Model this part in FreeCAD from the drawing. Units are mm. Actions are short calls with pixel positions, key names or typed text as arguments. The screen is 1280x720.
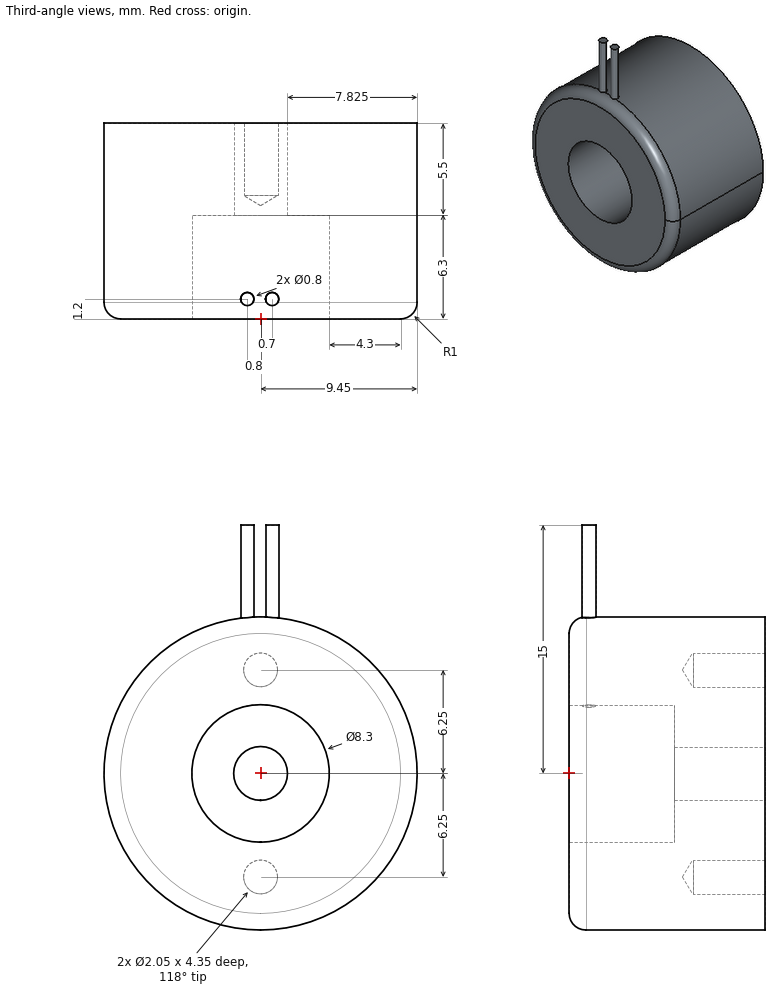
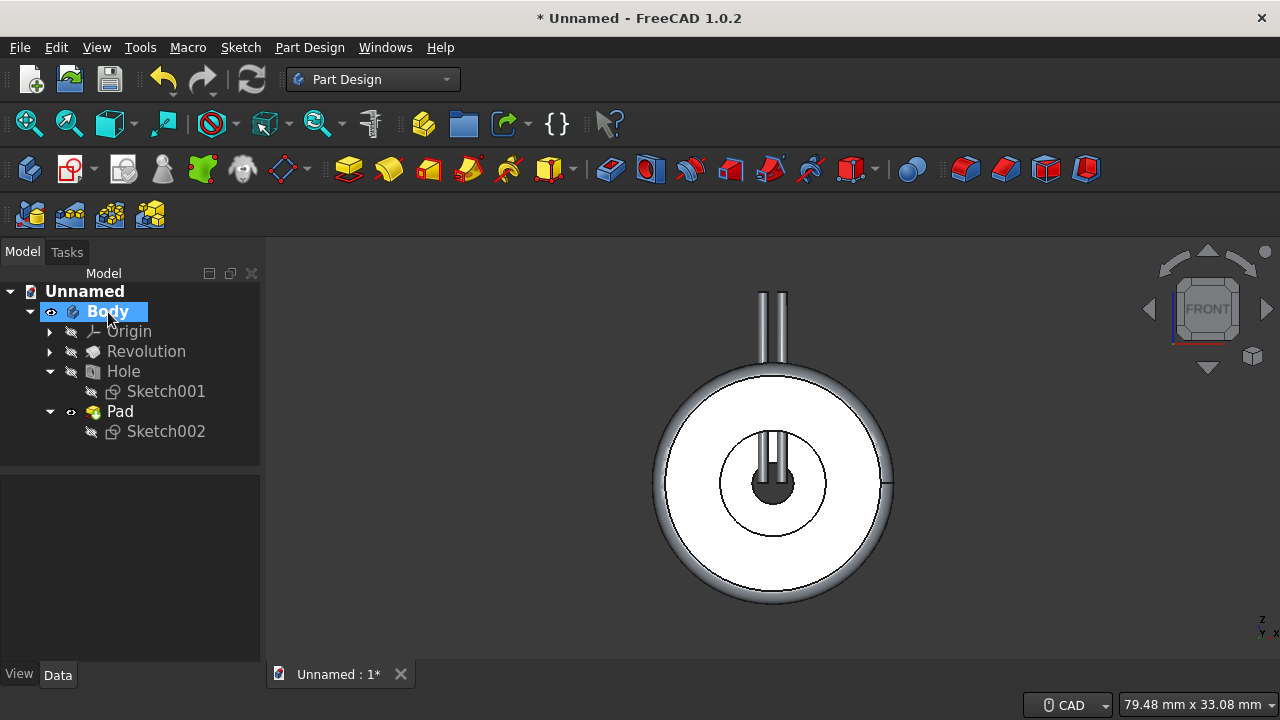
click(803, 498)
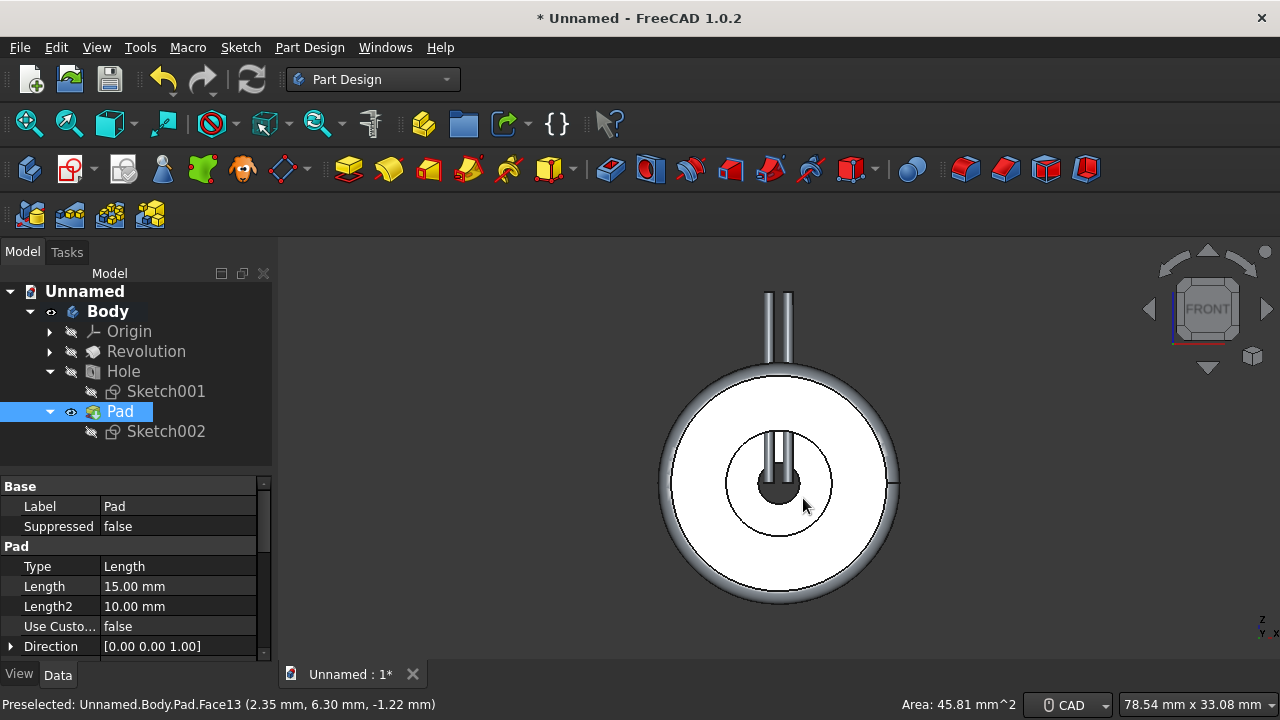
click(70, 170)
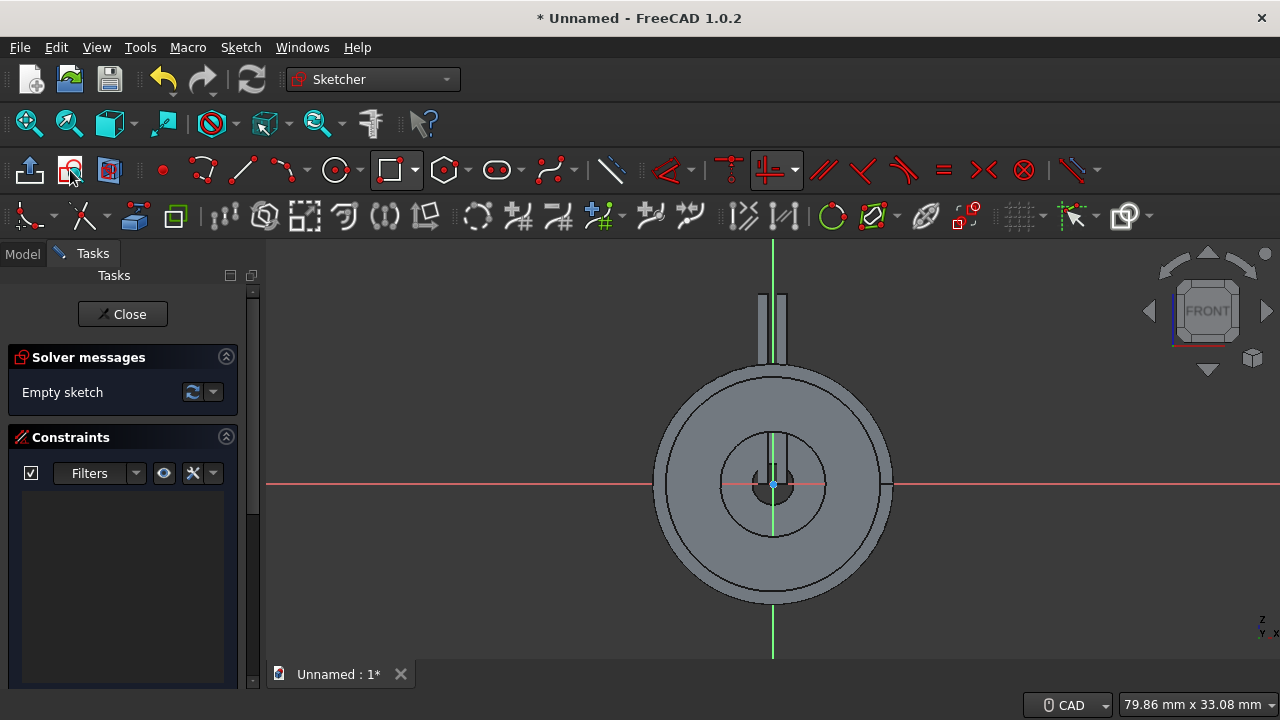
key(q)
key(s)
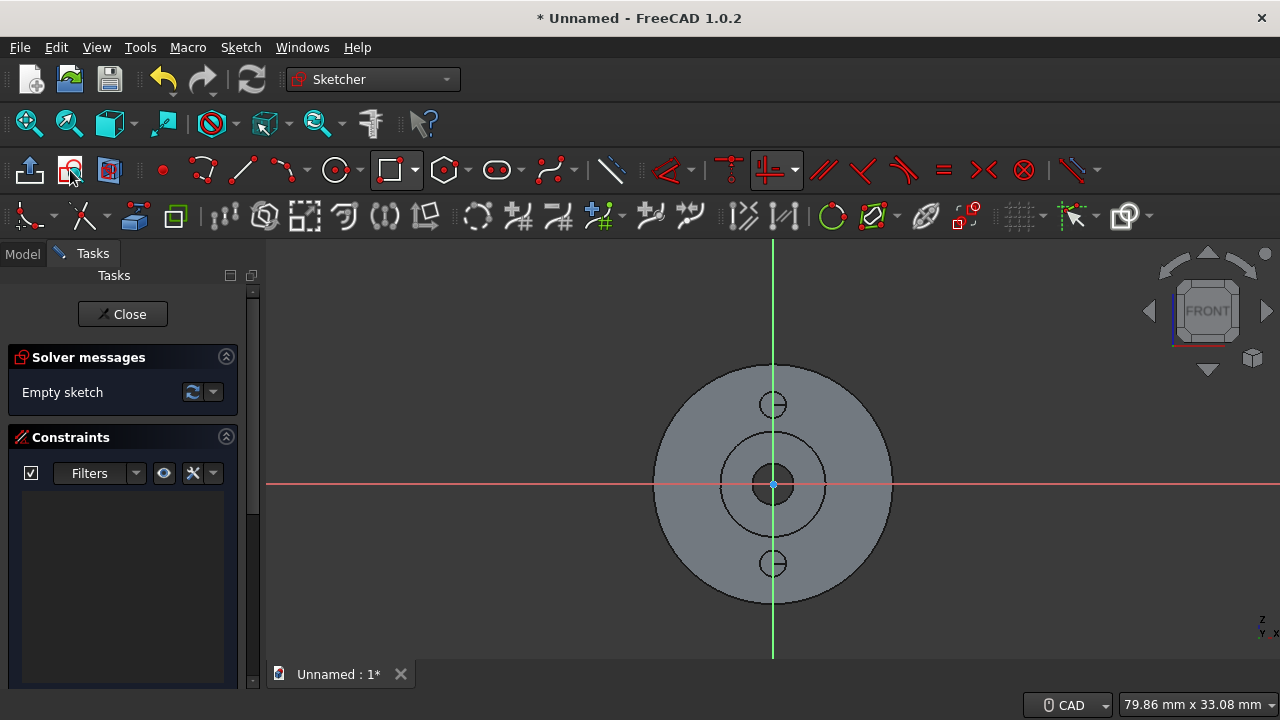
scroll(829, 513, up, 4)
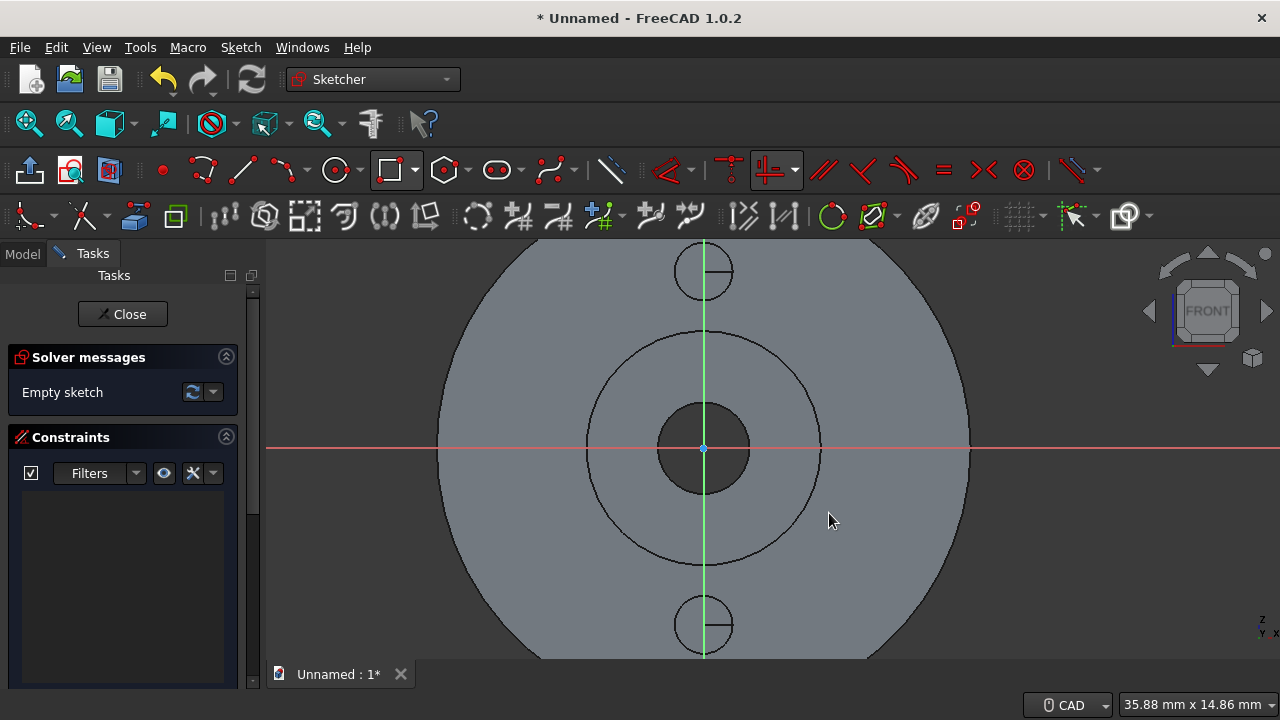
key(g)
key(c)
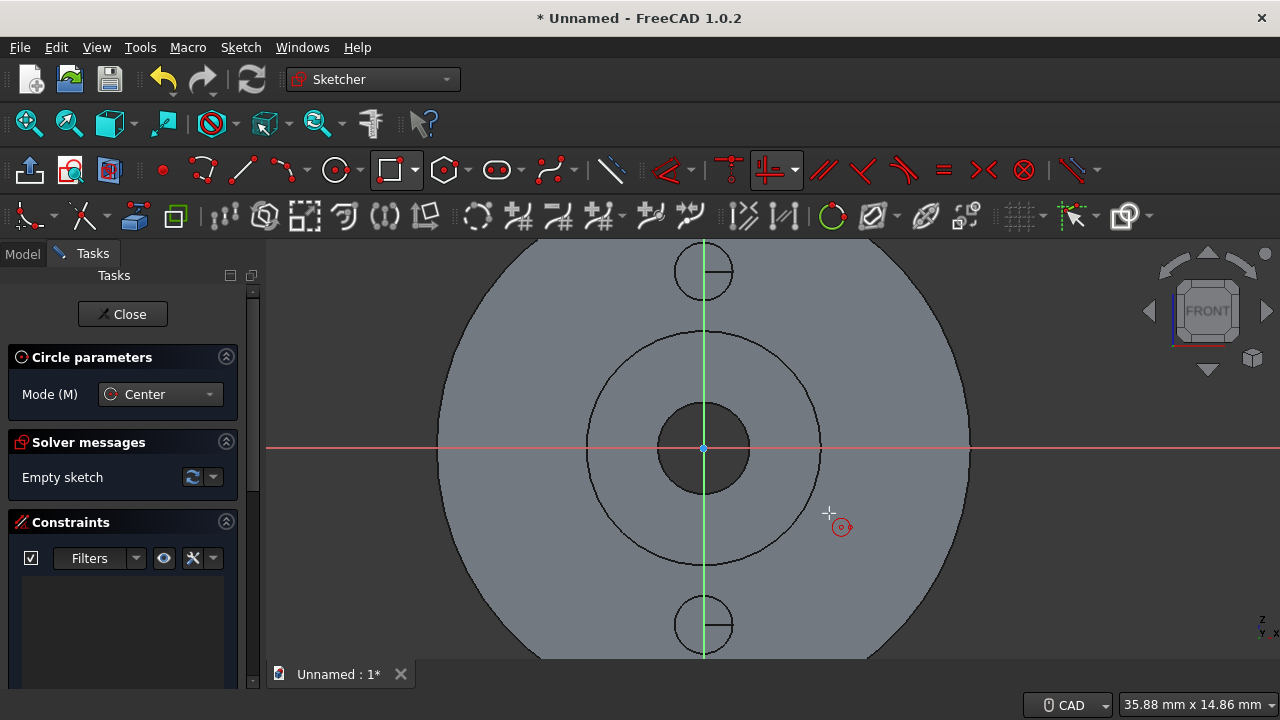
click(704, 448)
move(787, 365)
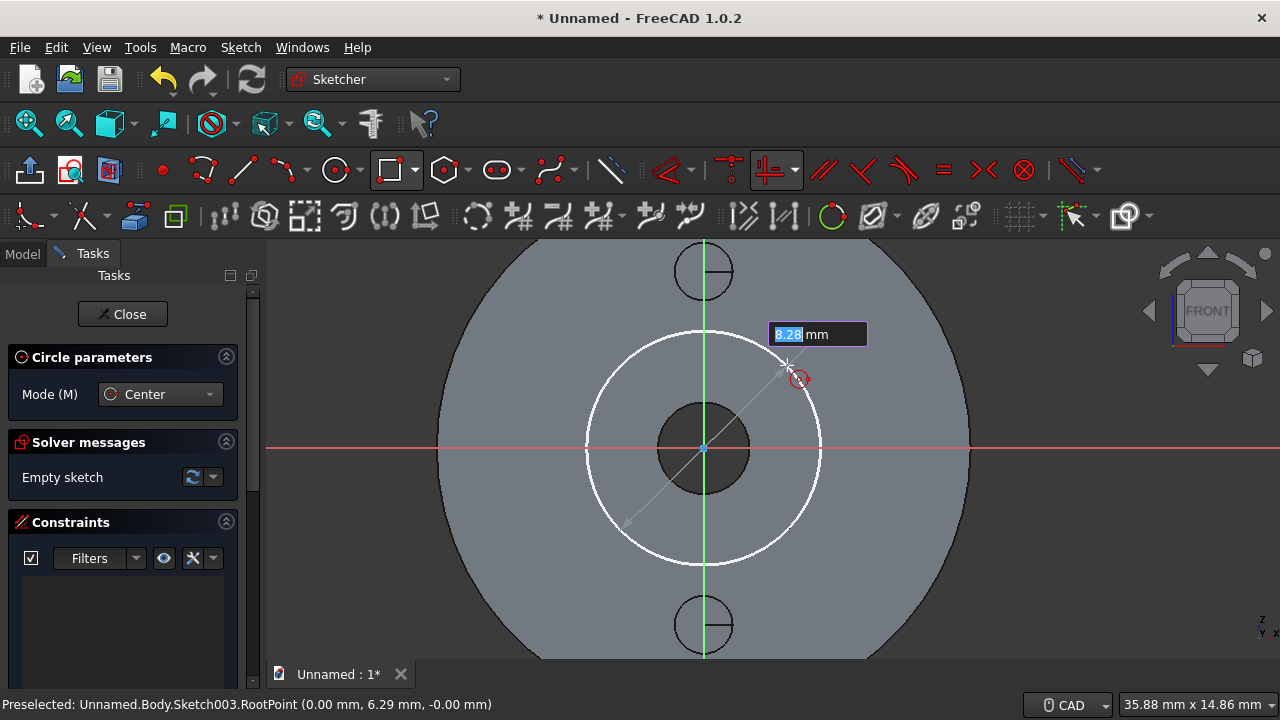
text(8.3)
key(Return)
key(Escape)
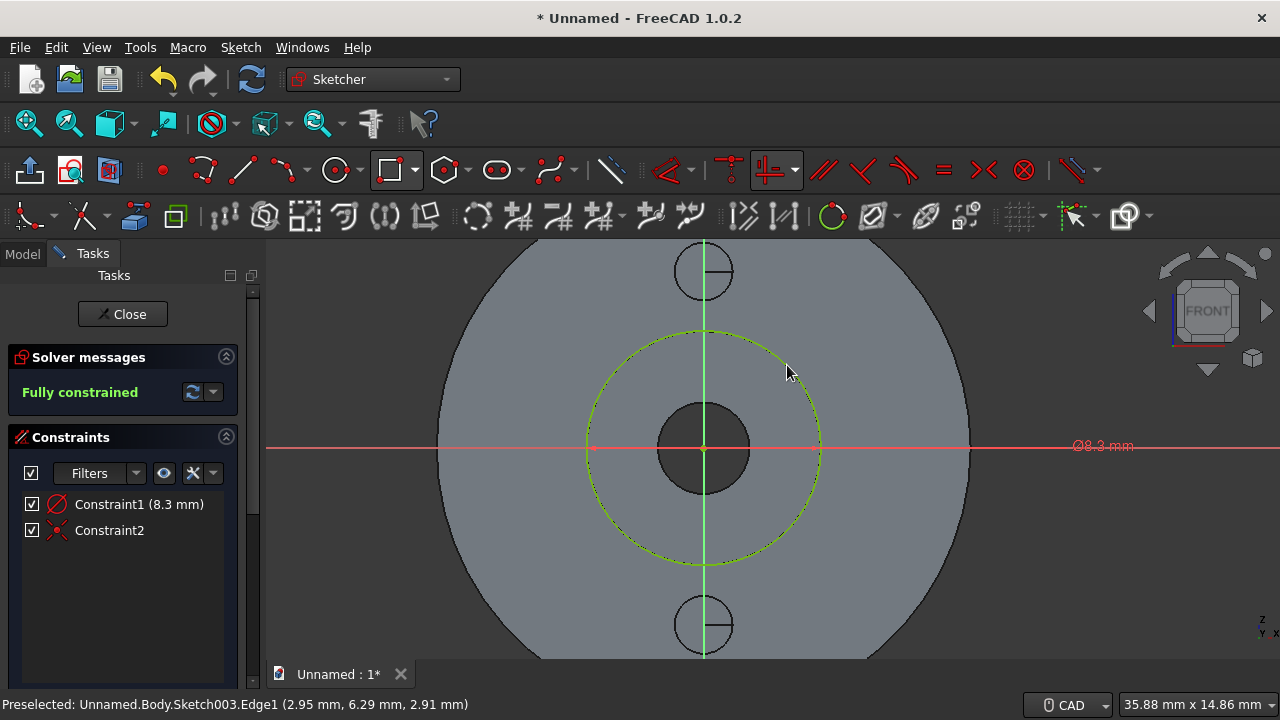
click(123, 314)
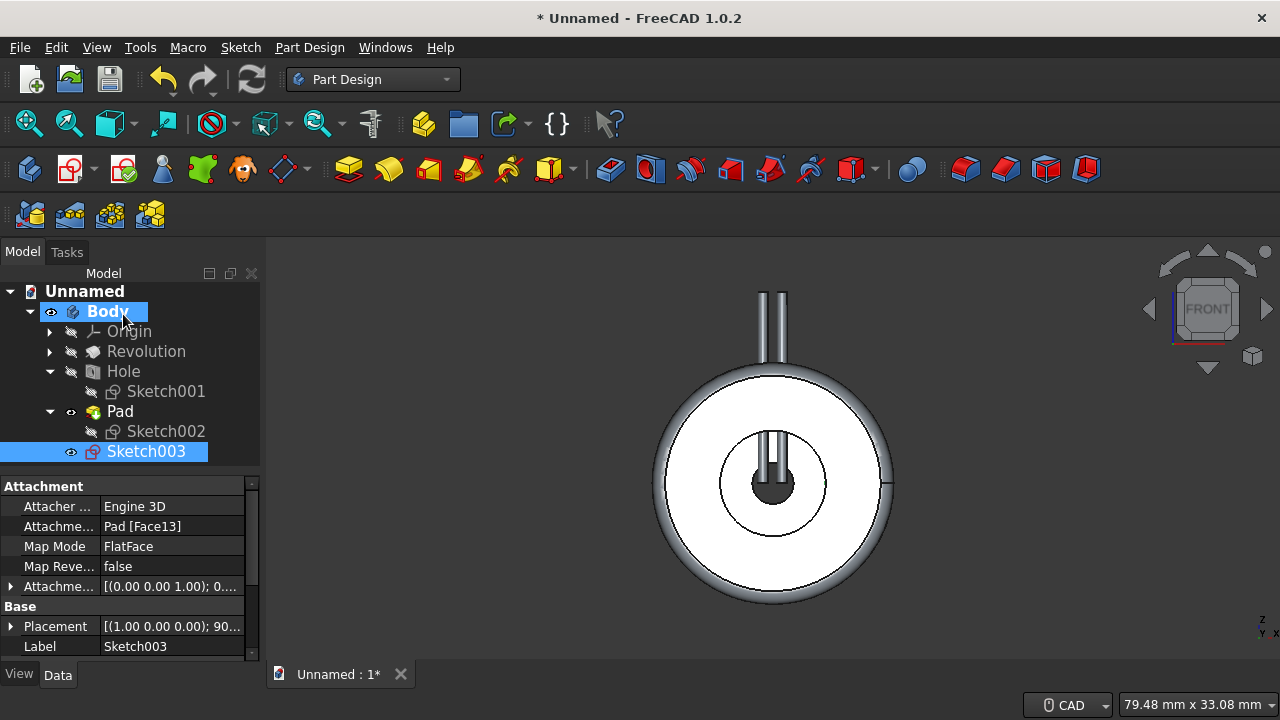
click(612, 170)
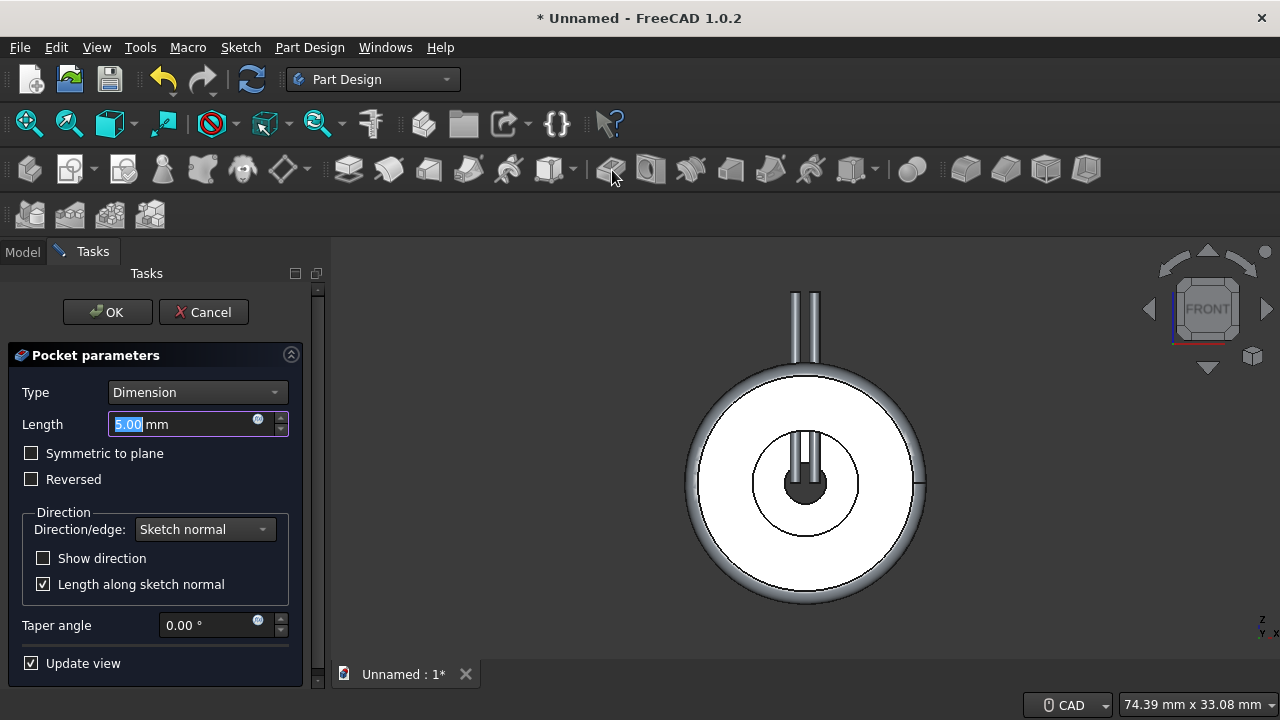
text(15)
key(Tab)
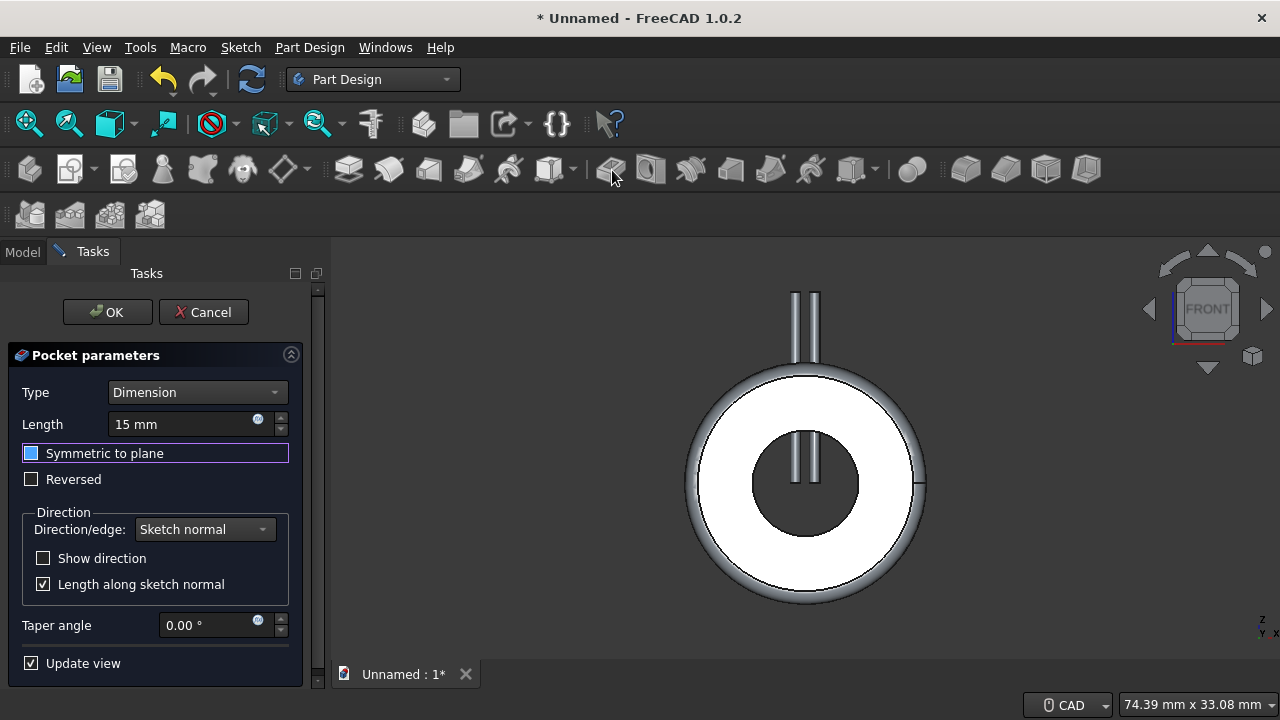
click(30, 479)